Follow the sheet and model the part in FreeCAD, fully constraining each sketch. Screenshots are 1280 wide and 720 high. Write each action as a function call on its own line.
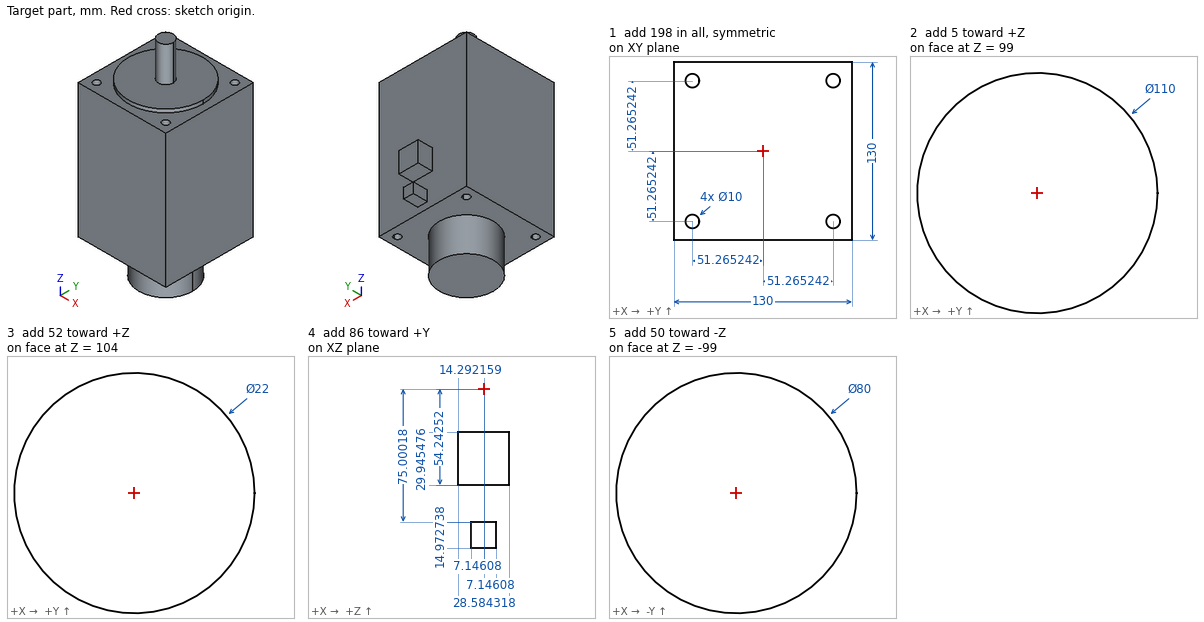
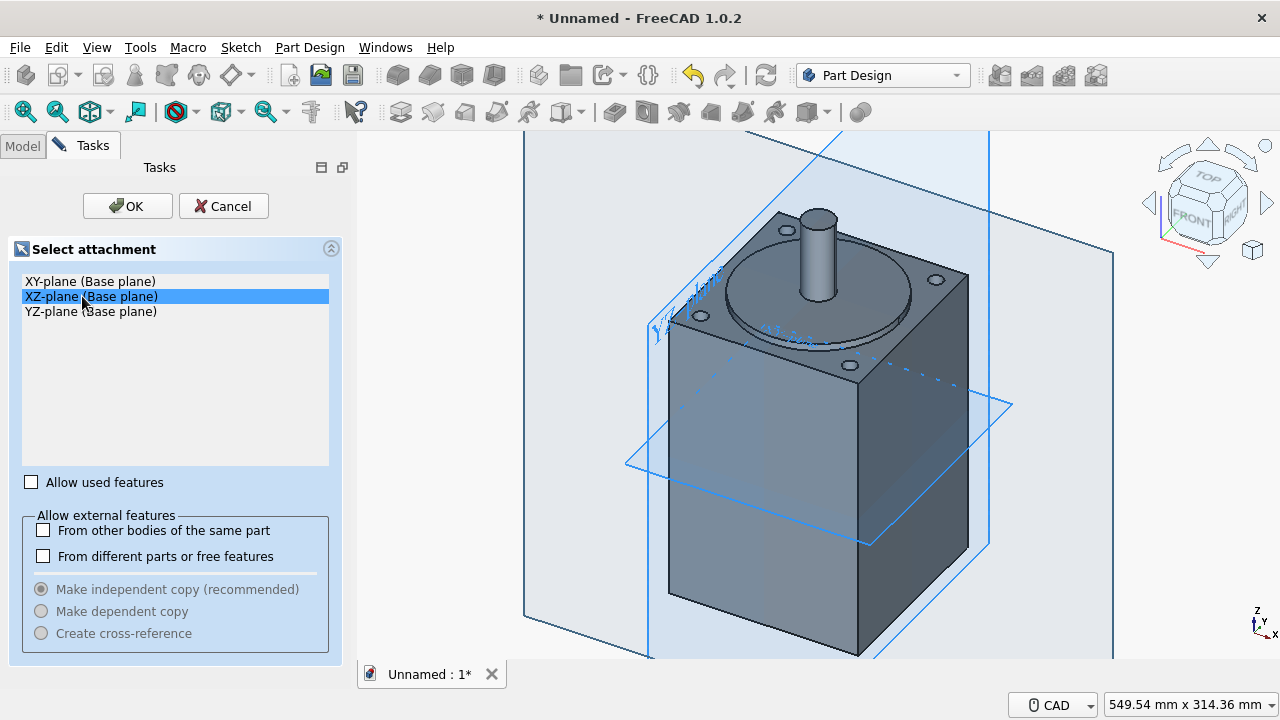
click(128, 206)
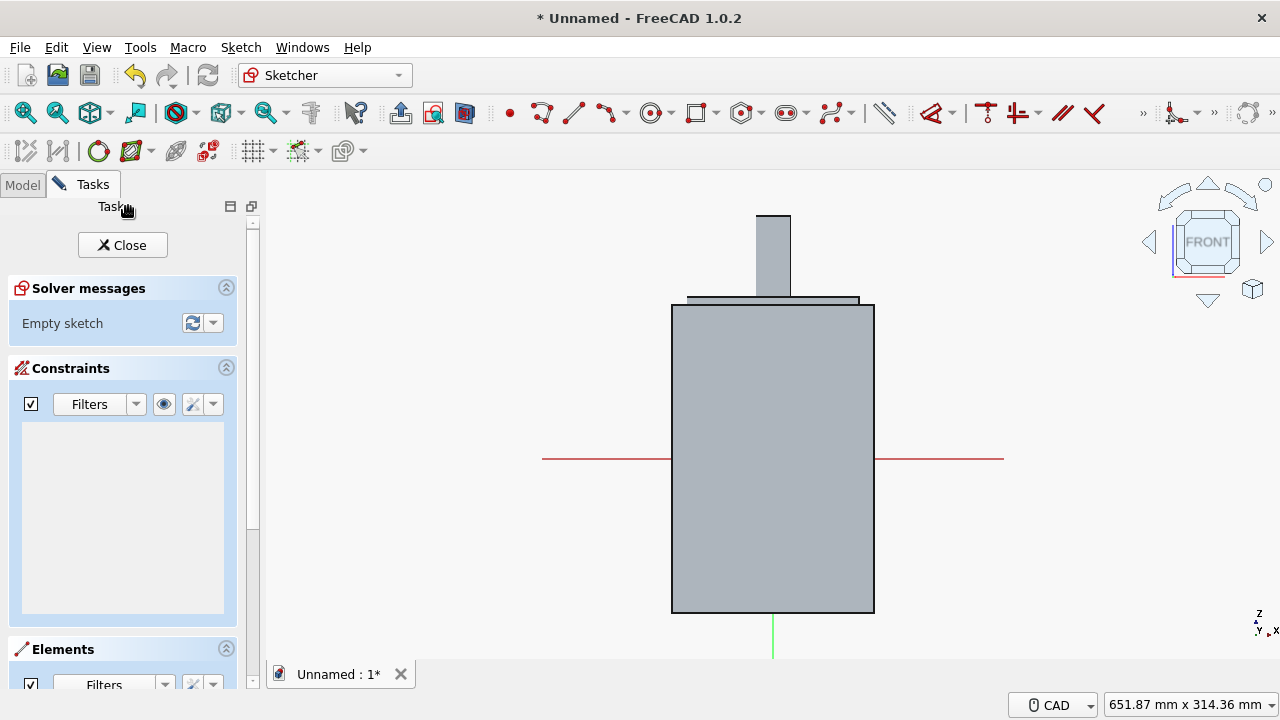
key(q)
key(s)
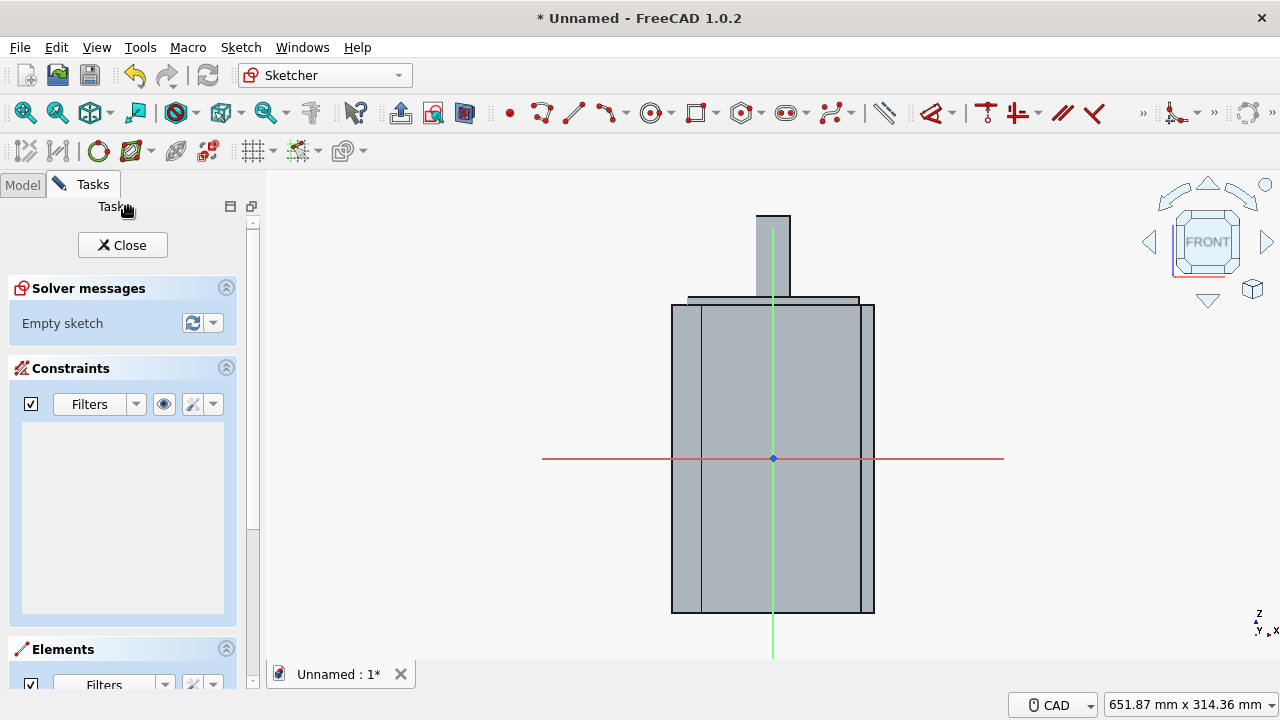
scroll(829, 622, up, 4)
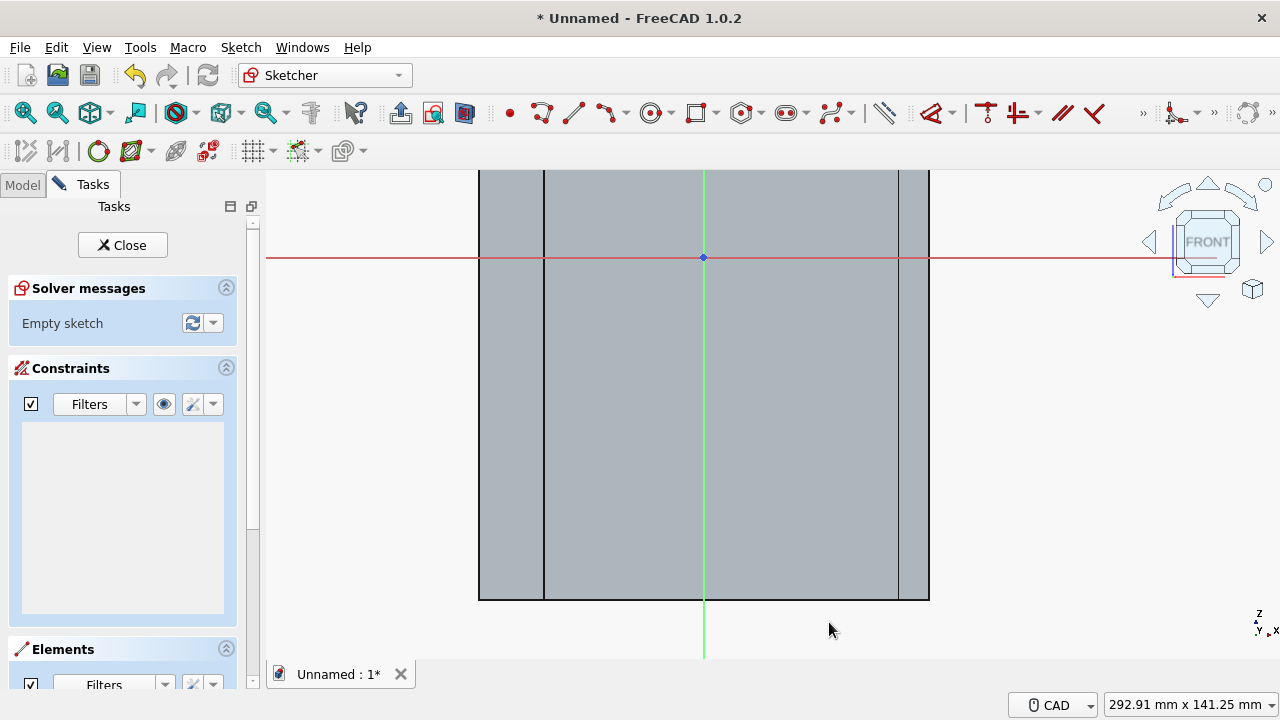
key(g)
key(r)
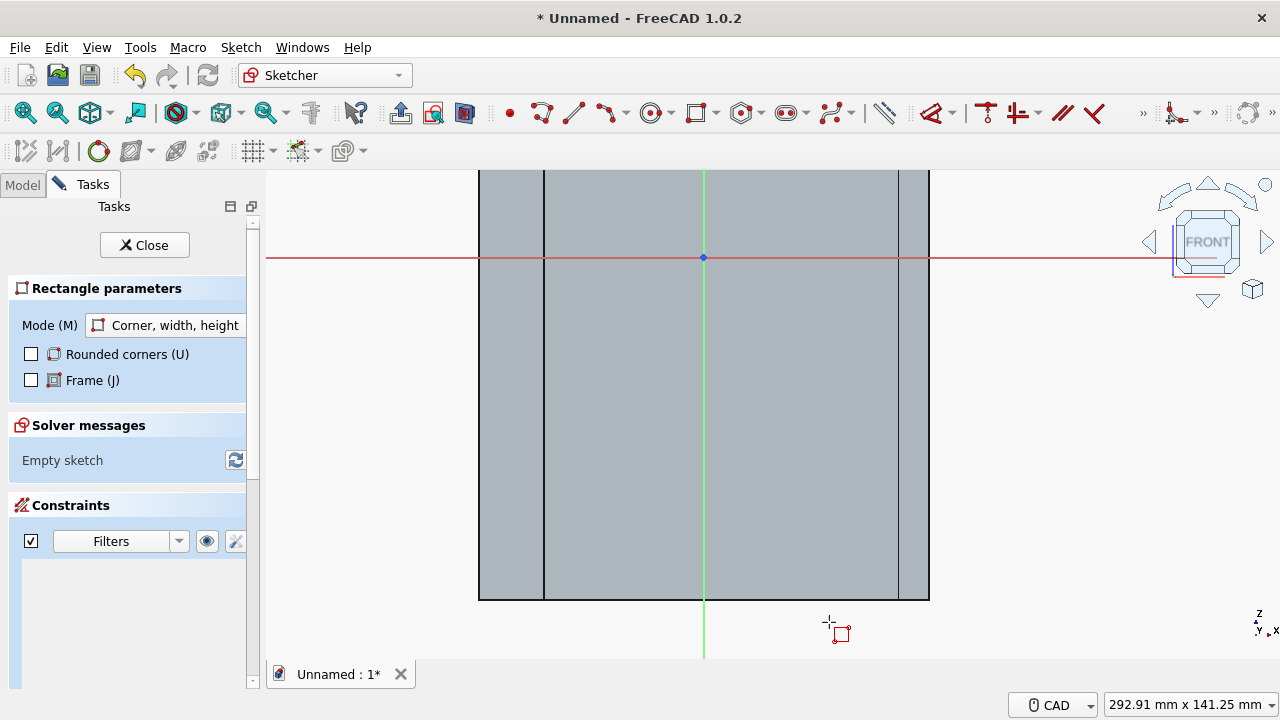
click(654, 342)
click(753, 446)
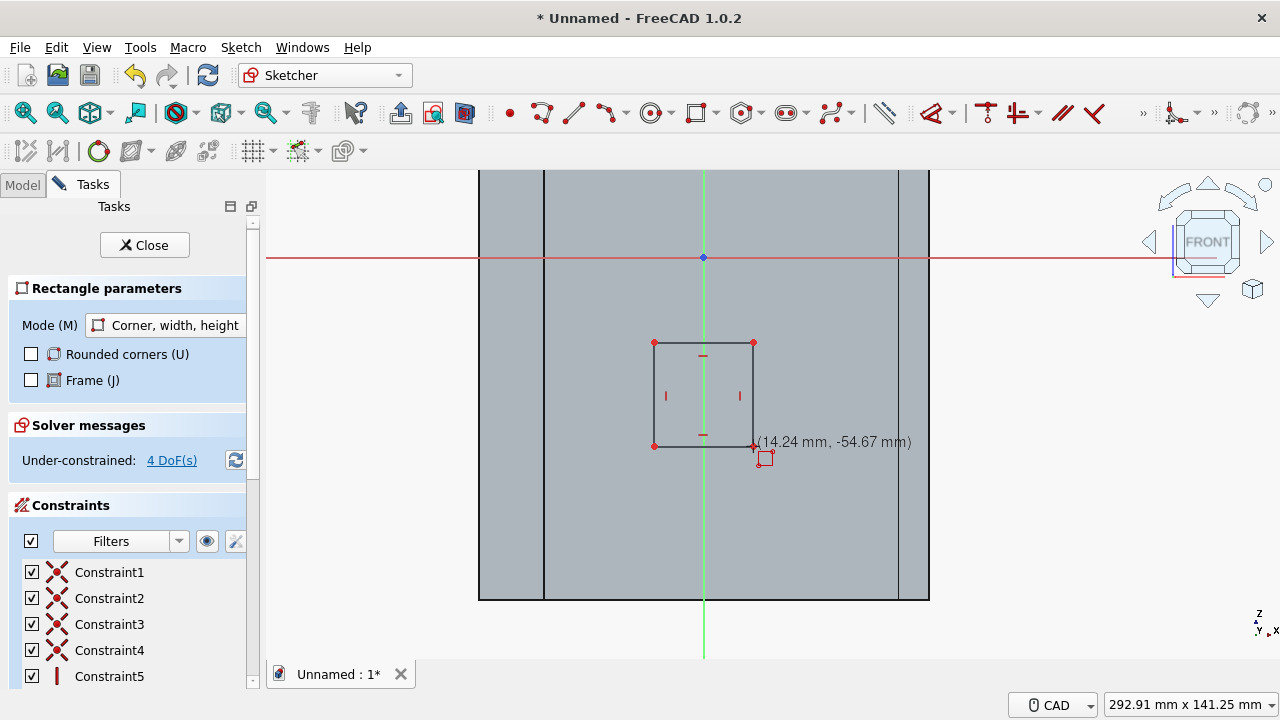
click(679, 517)
click(728, 569)
key(Escape)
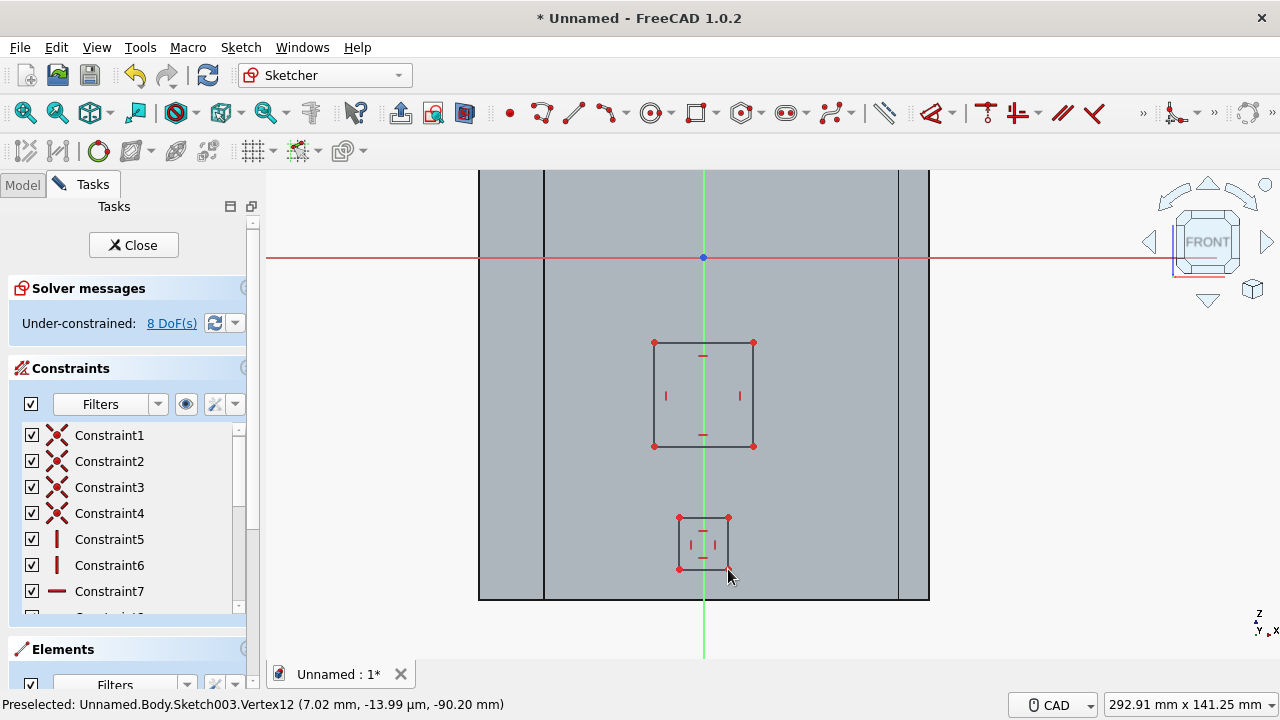
click(932, 114)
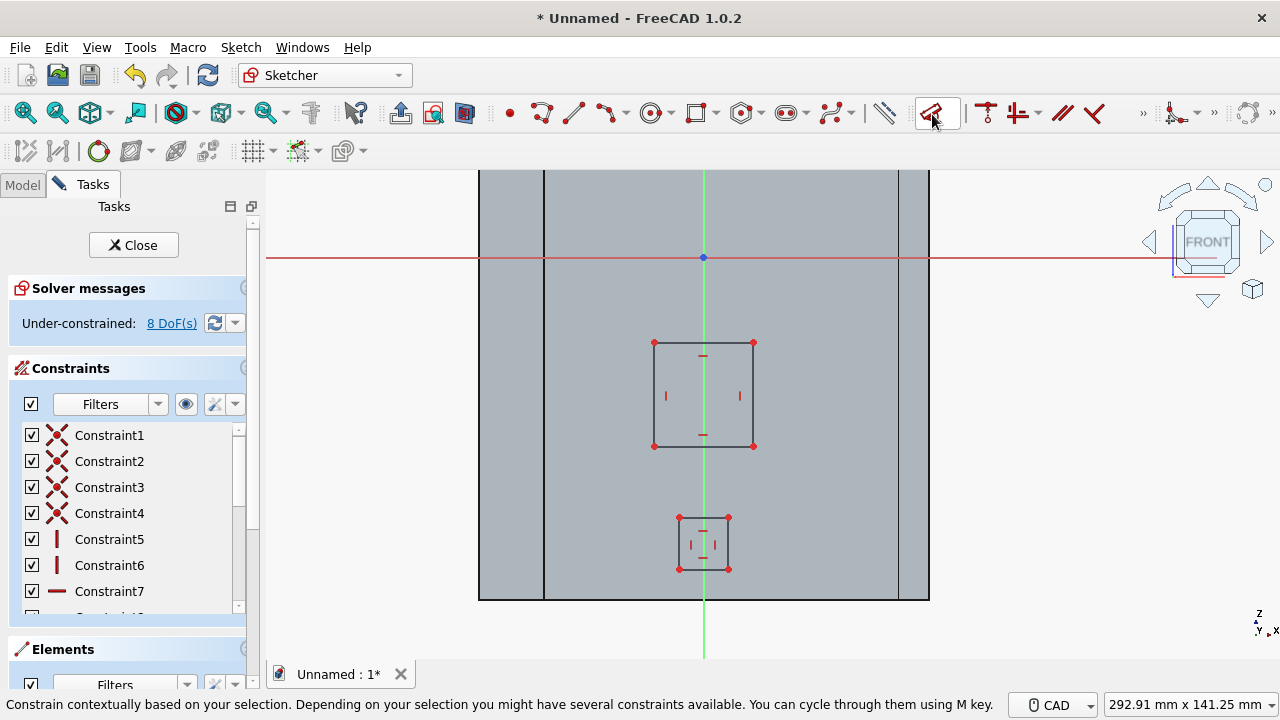
scroll(679, 518, up, 3)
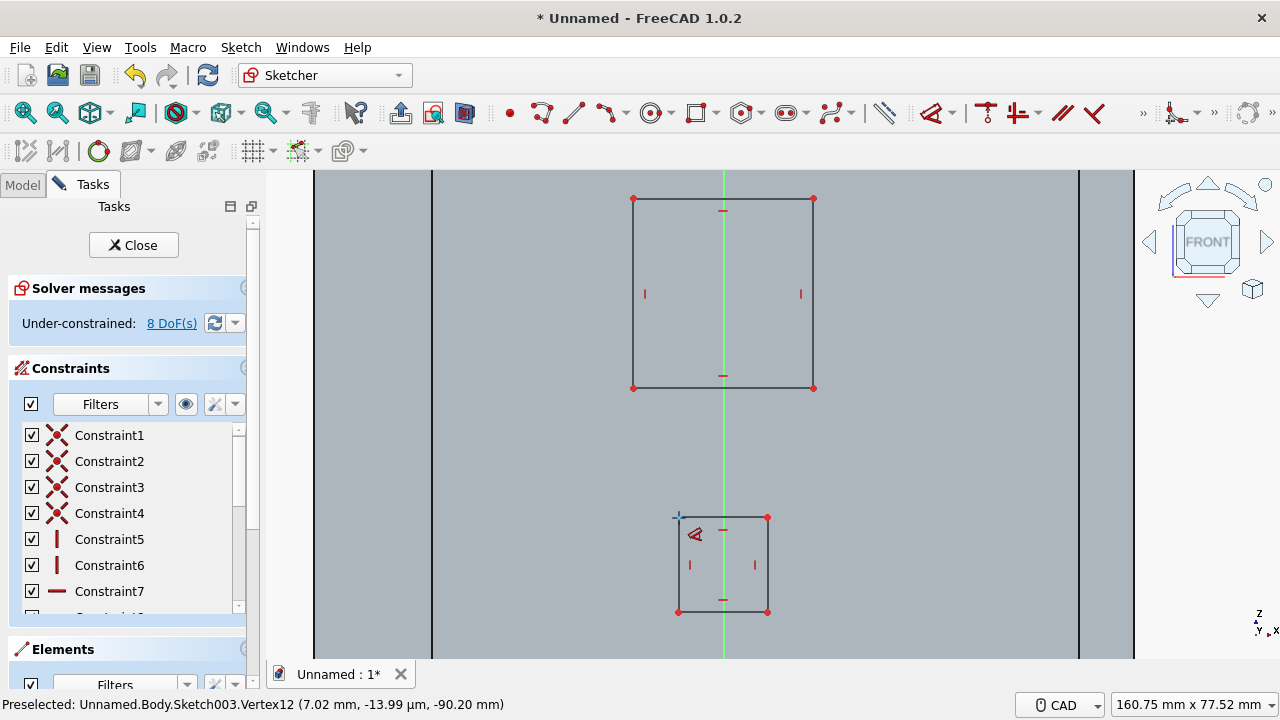
click(679, 517)
click(701, 551)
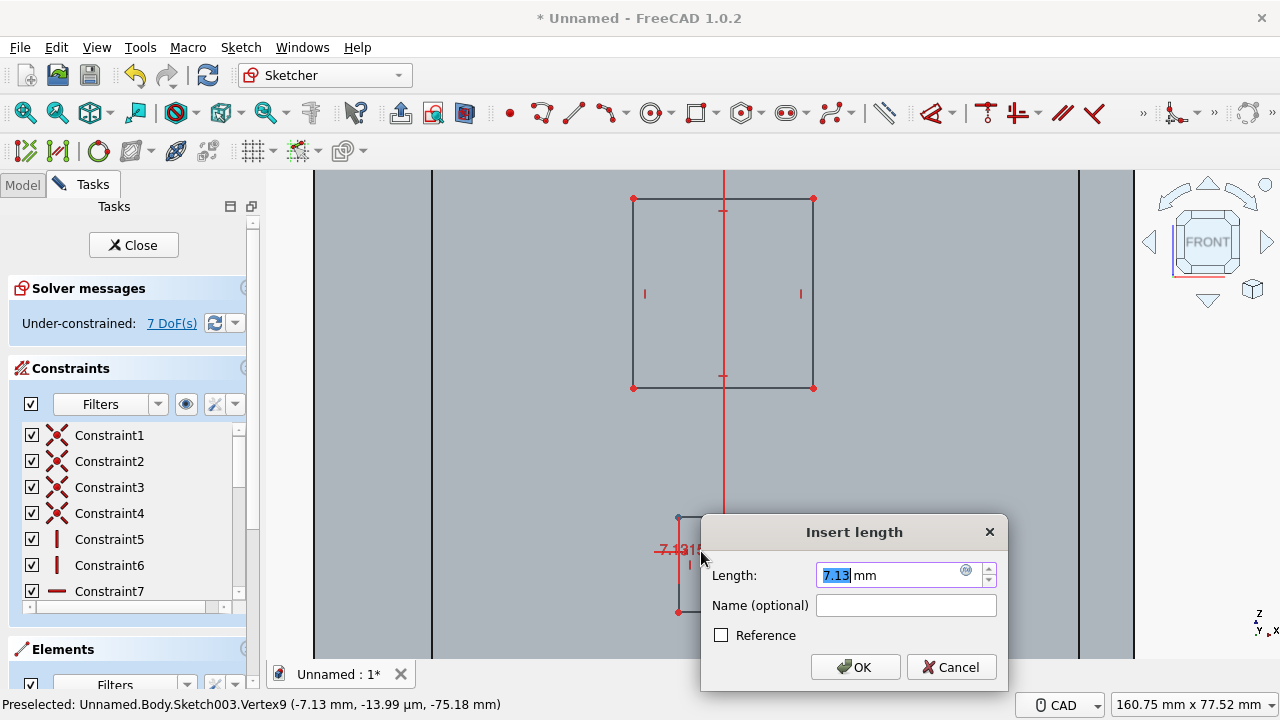
text(7.14608)
key(Return)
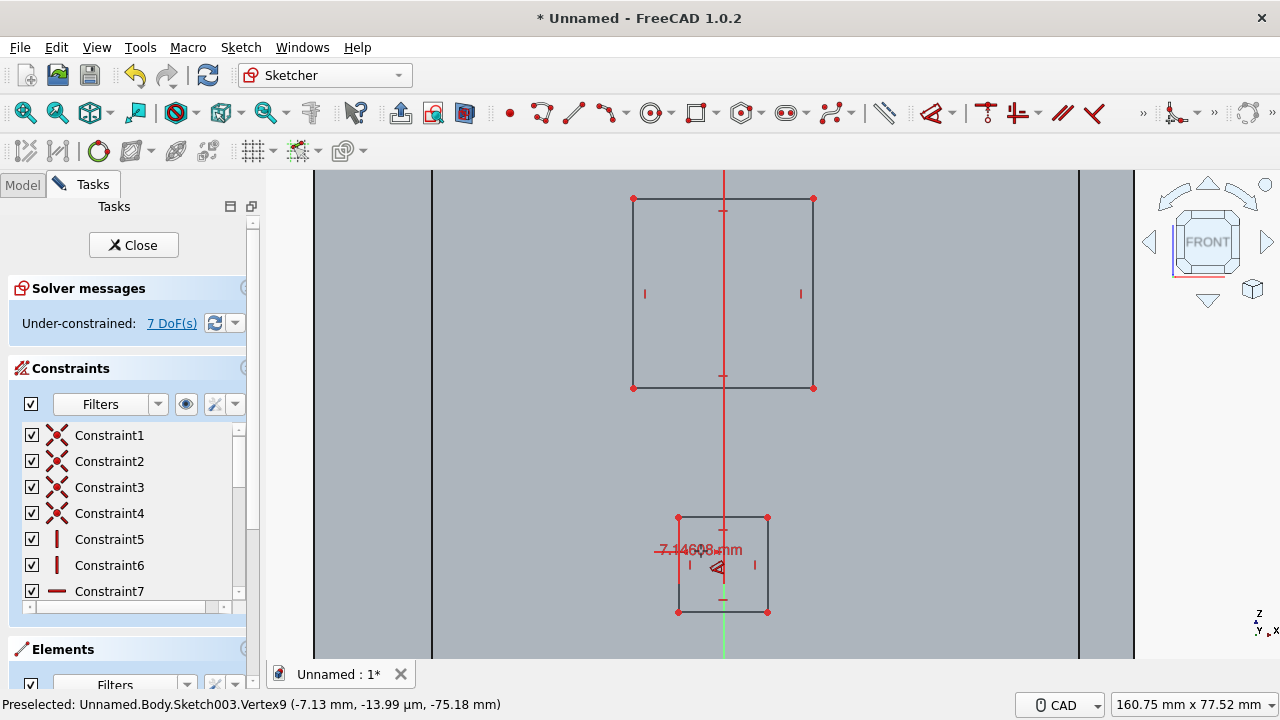
click(768, 612)